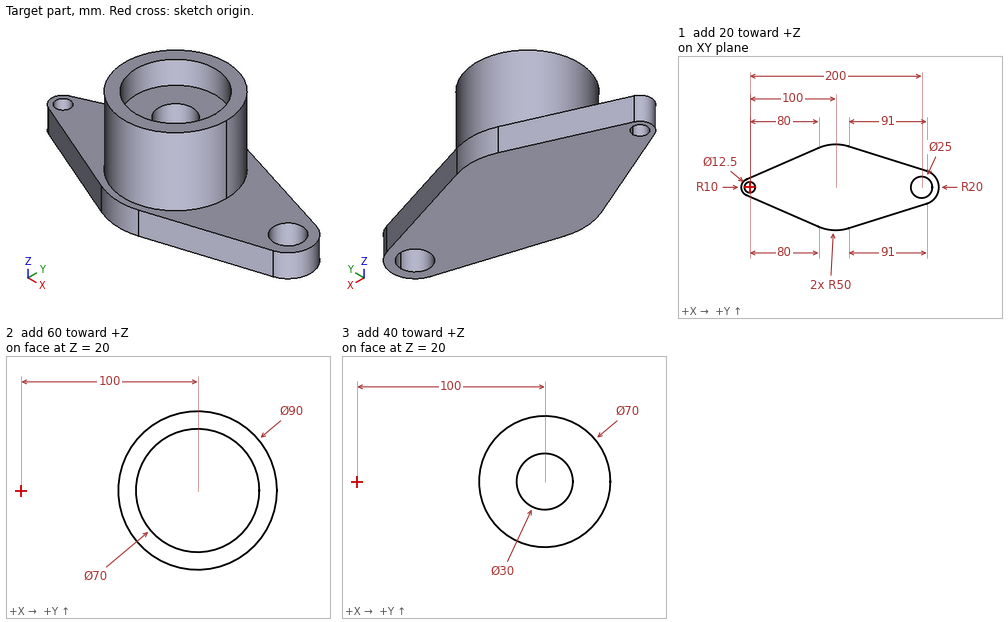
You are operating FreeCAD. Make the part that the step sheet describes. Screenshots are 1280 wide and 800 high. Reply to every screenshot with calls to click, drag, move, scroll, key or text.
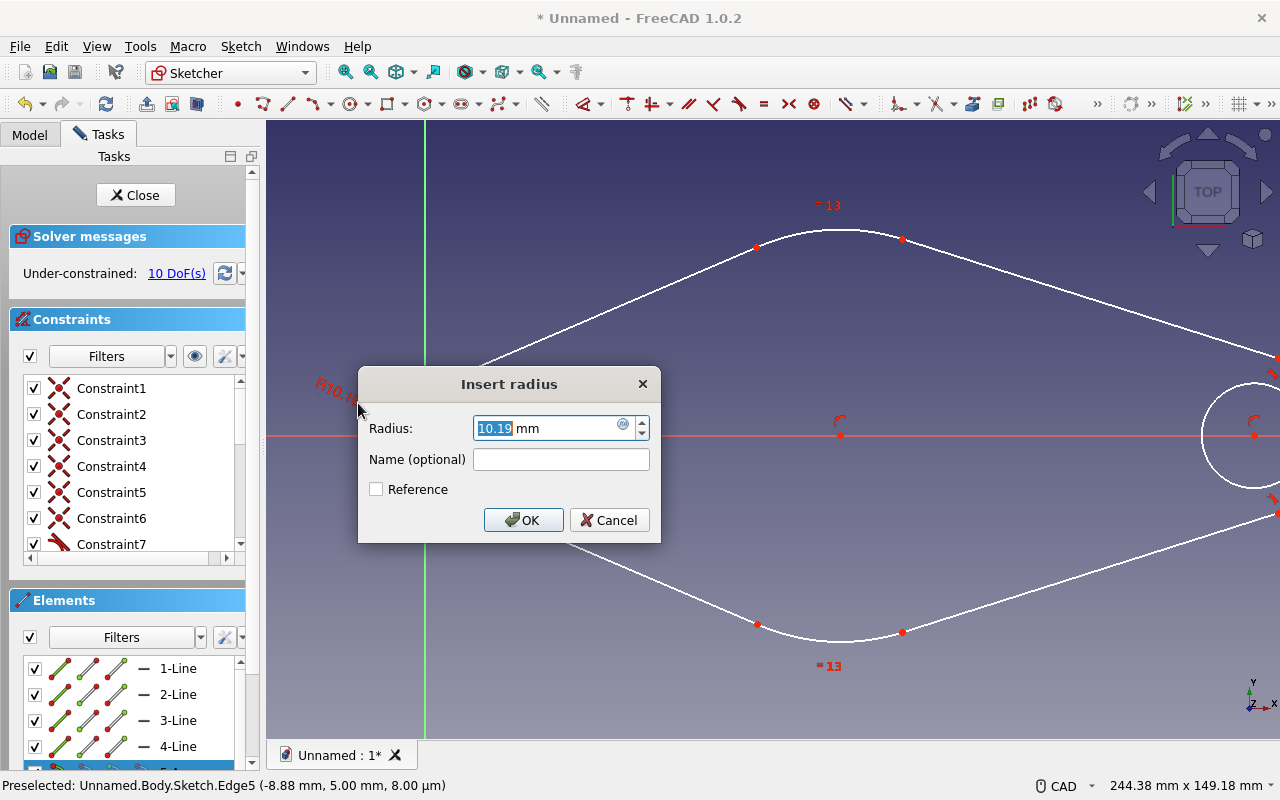
text(10)
key(Return)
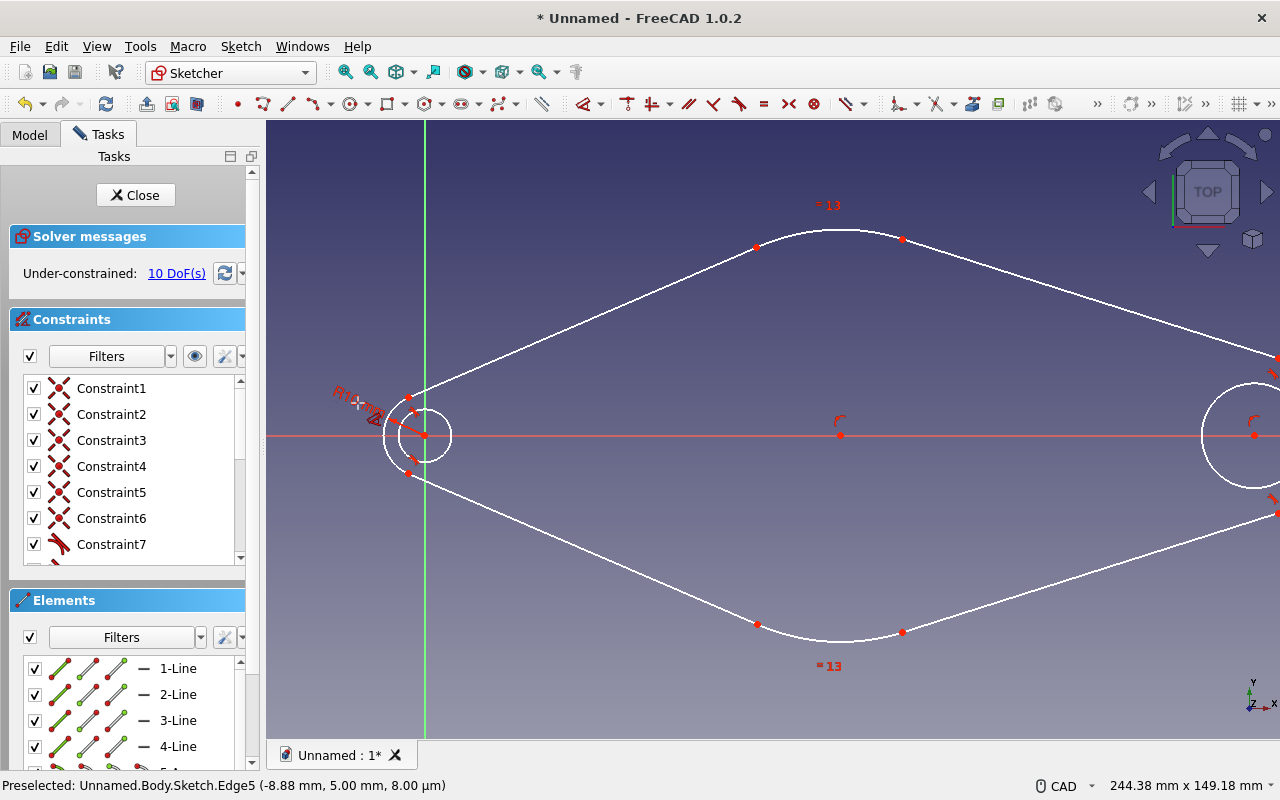
click(800, 638)
click(794, 669)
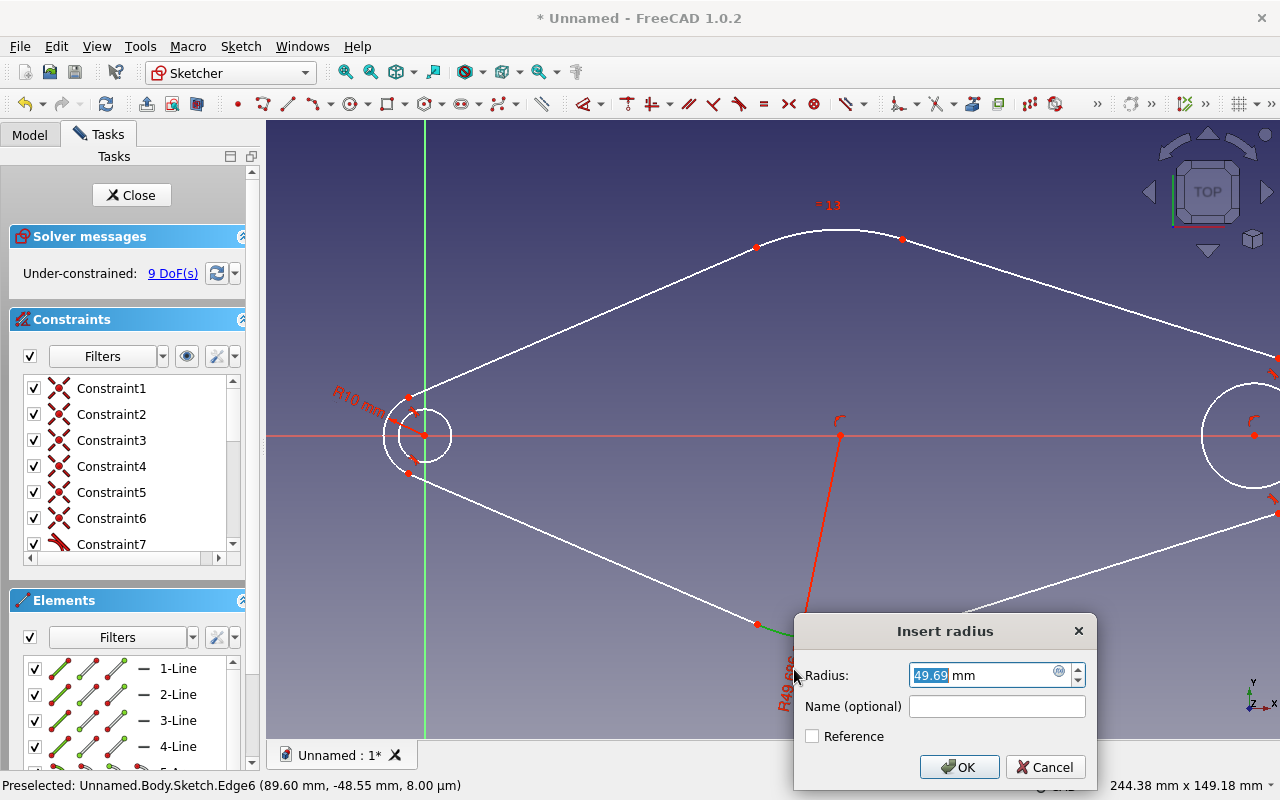
text(50)
key(Return)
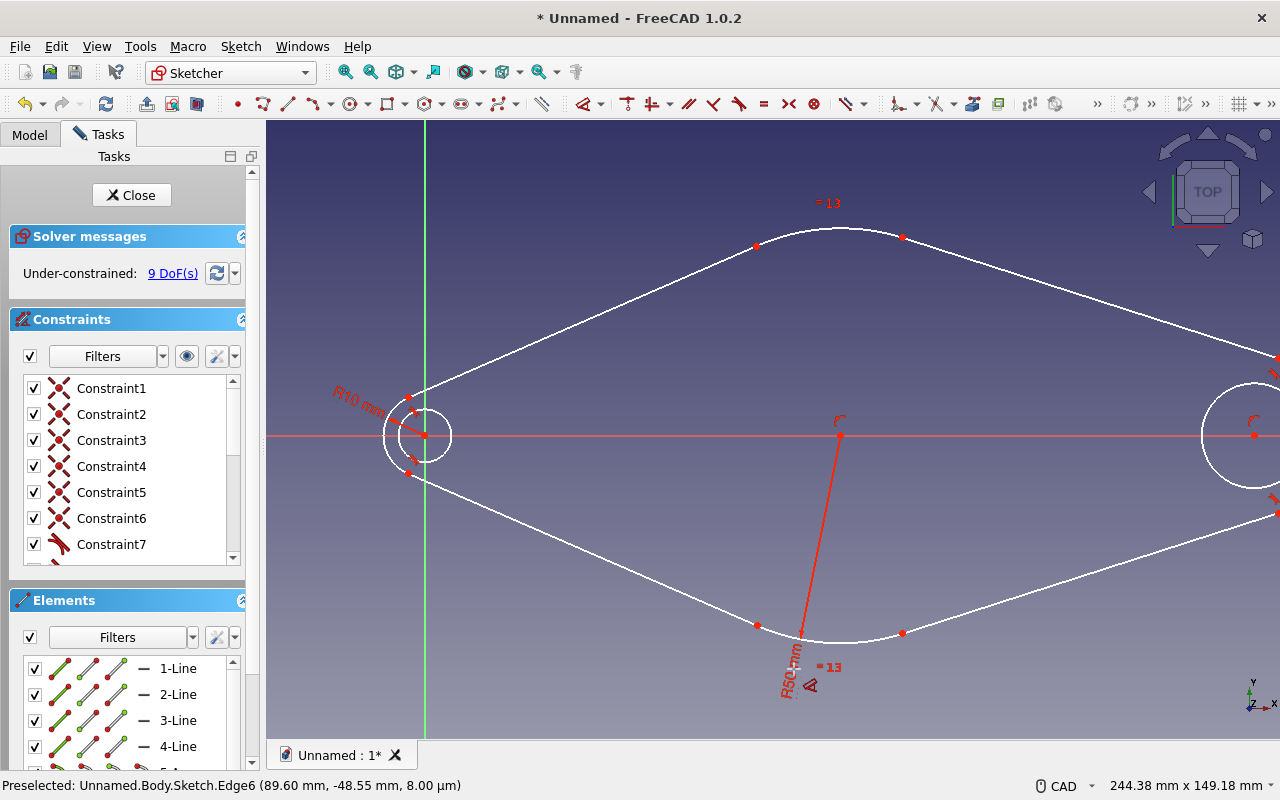
scroll(387, 417, down, 2)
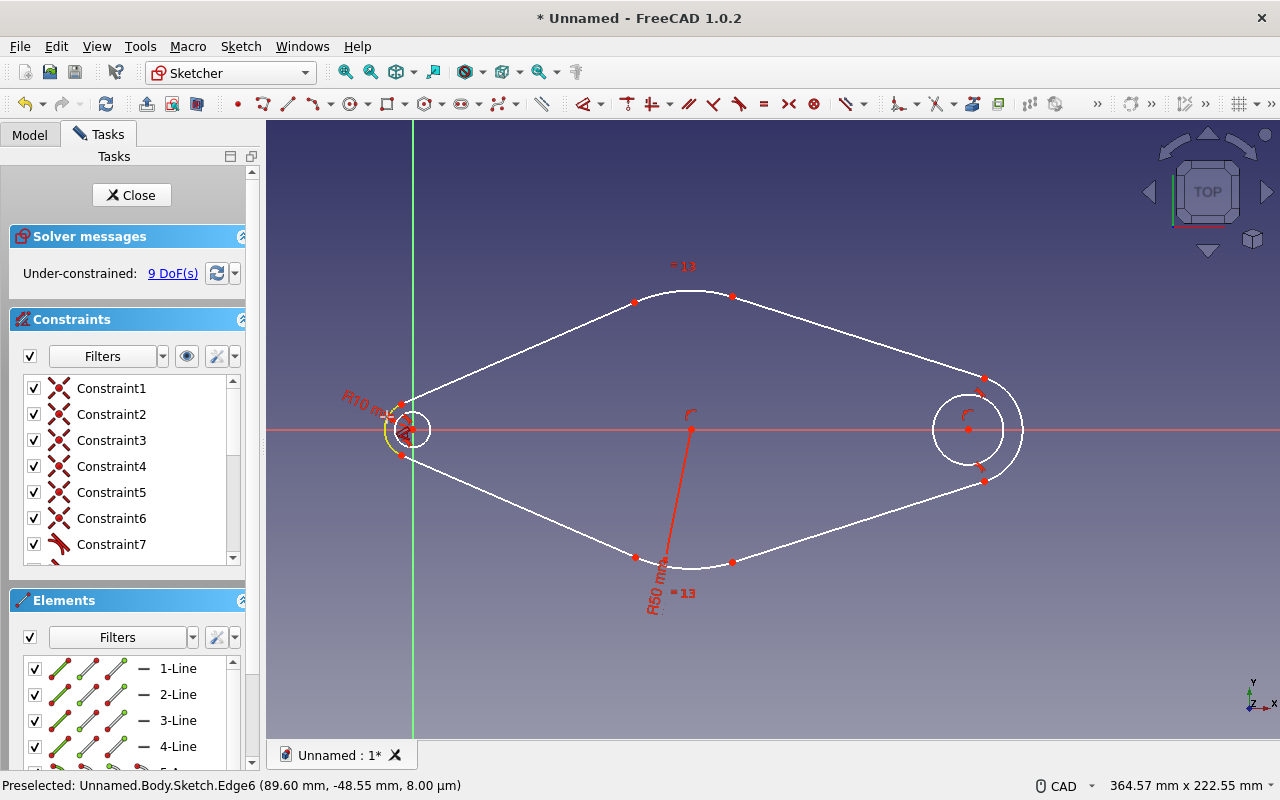
click(1016, 456)
click(1044, 471)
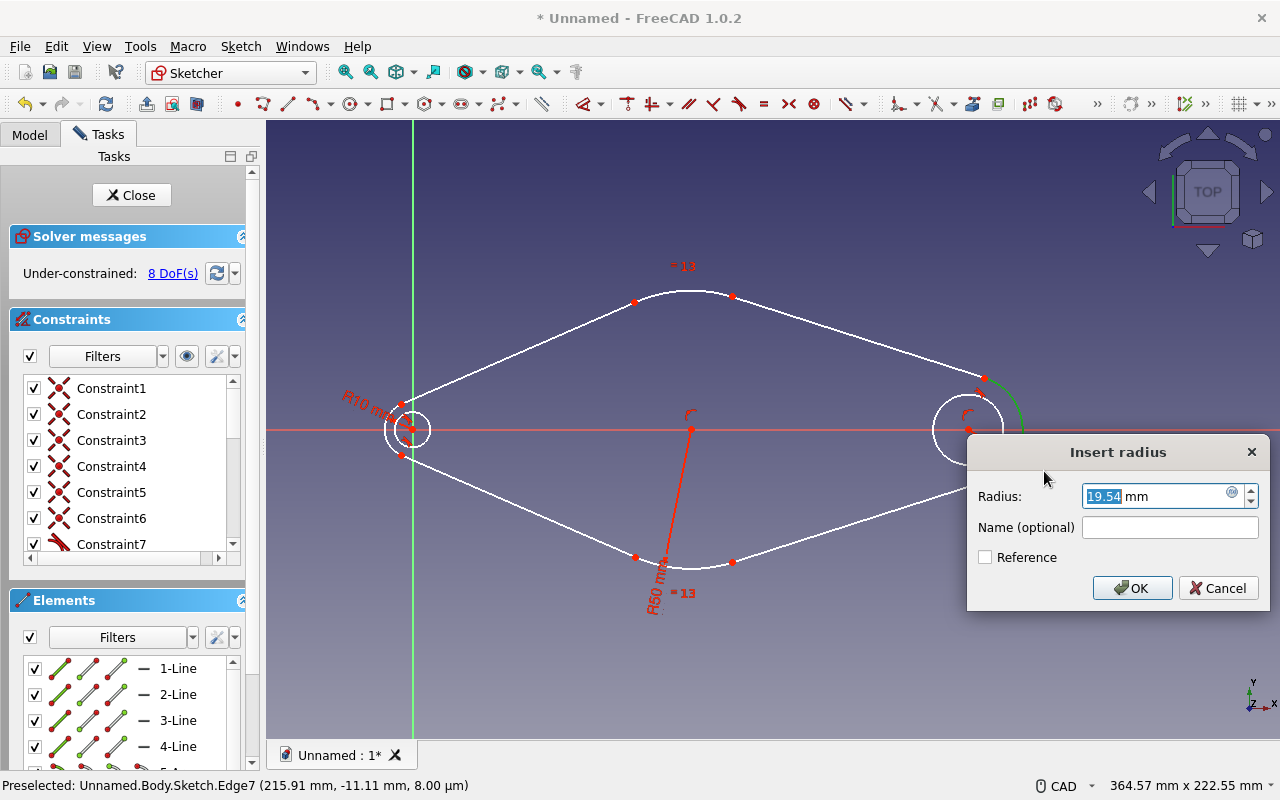
text(20)
key(Return)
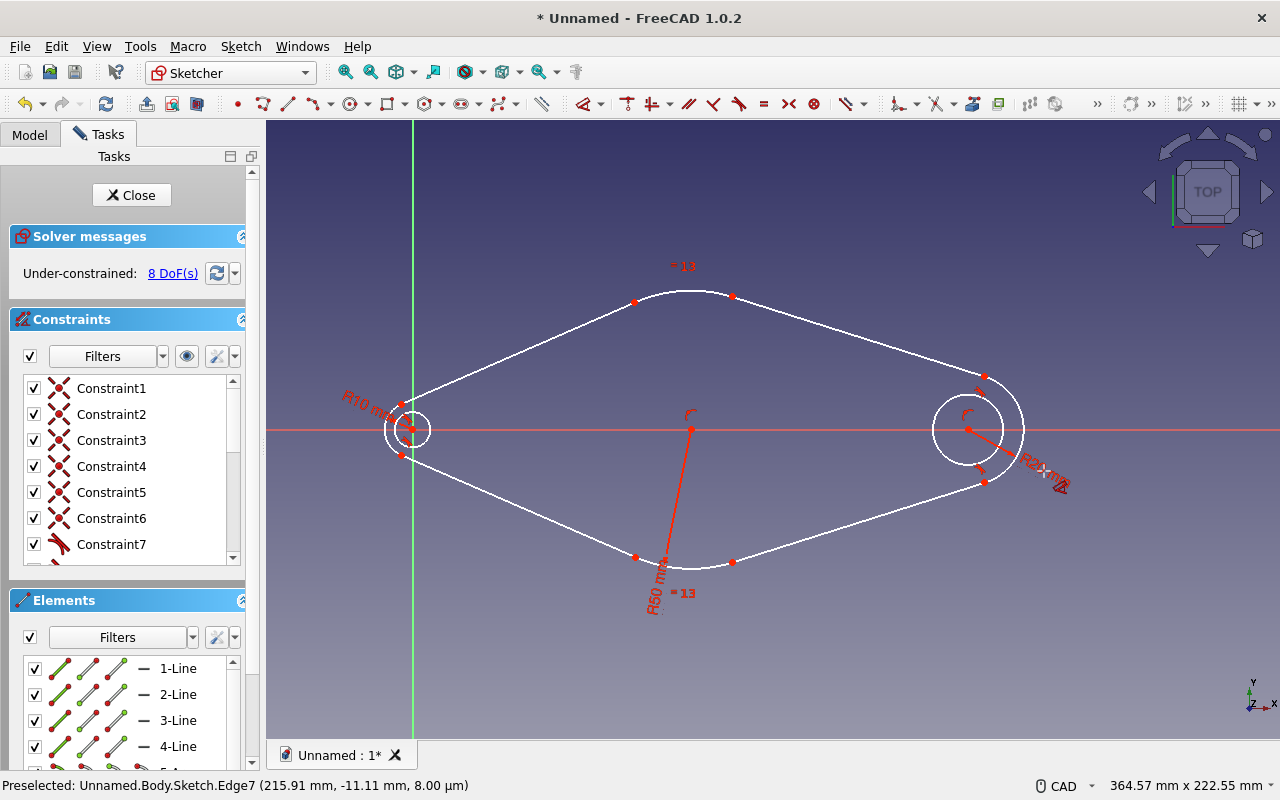
click(993, 405)
click(921, 382)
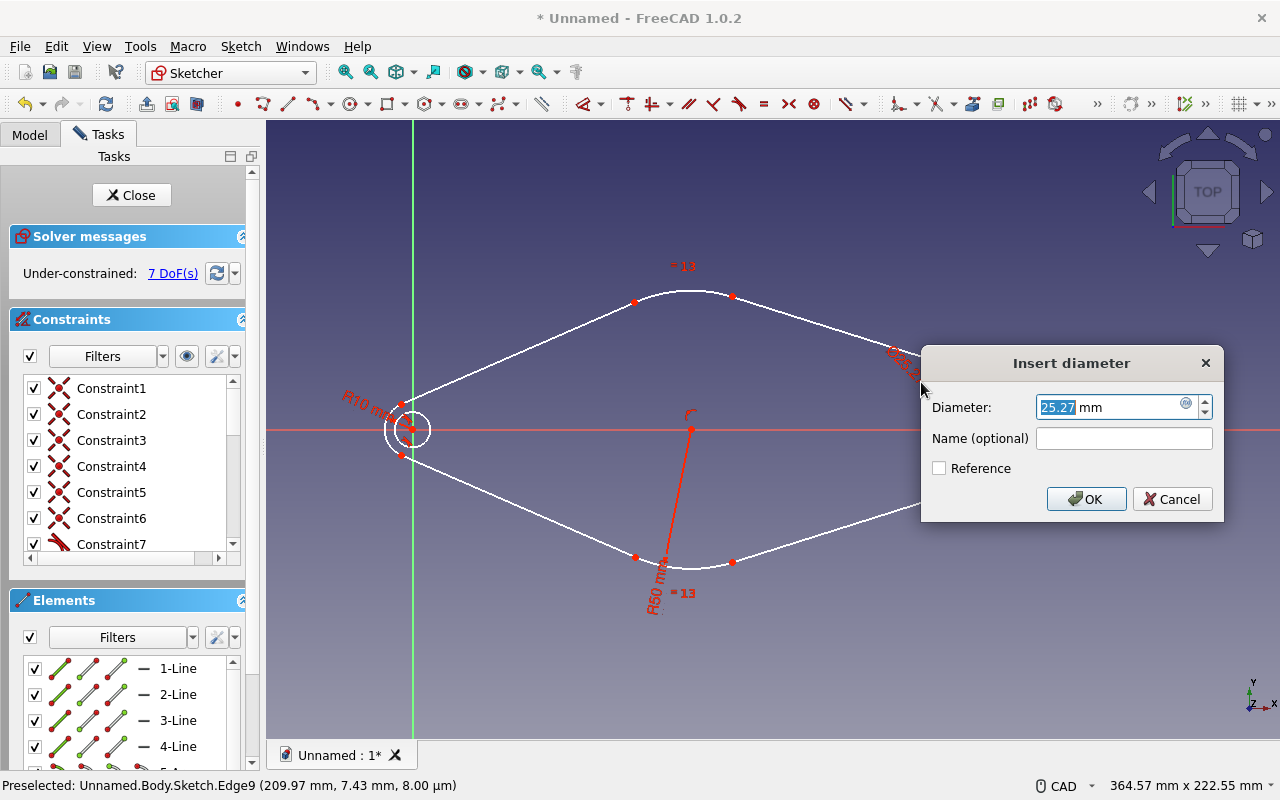
text(25)
key(Return)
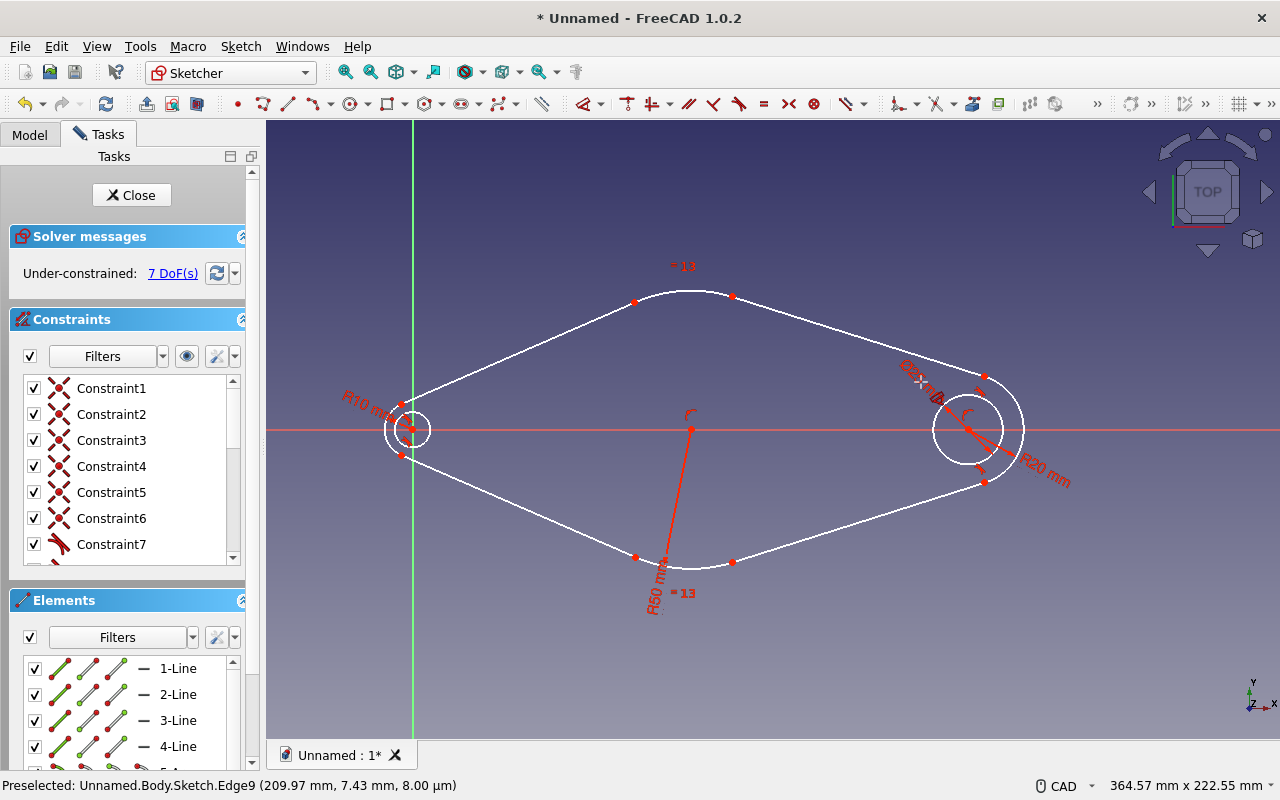
click(425, 417)
click(460, 415)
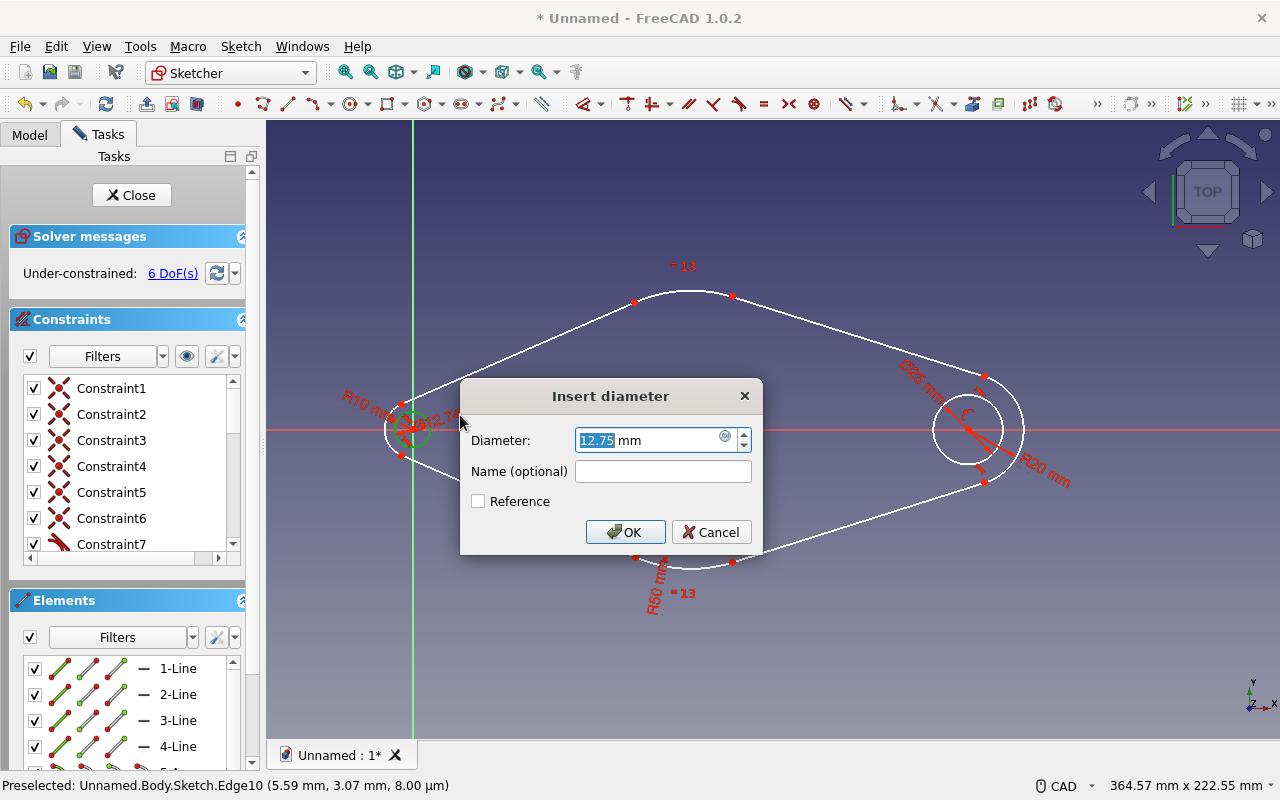
text(12.5)
key(Return)